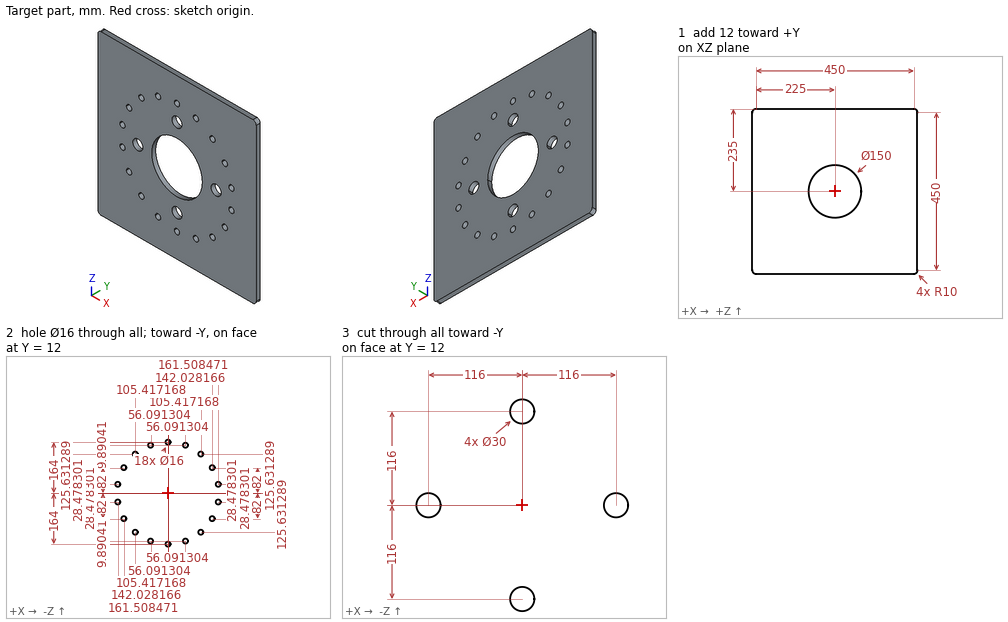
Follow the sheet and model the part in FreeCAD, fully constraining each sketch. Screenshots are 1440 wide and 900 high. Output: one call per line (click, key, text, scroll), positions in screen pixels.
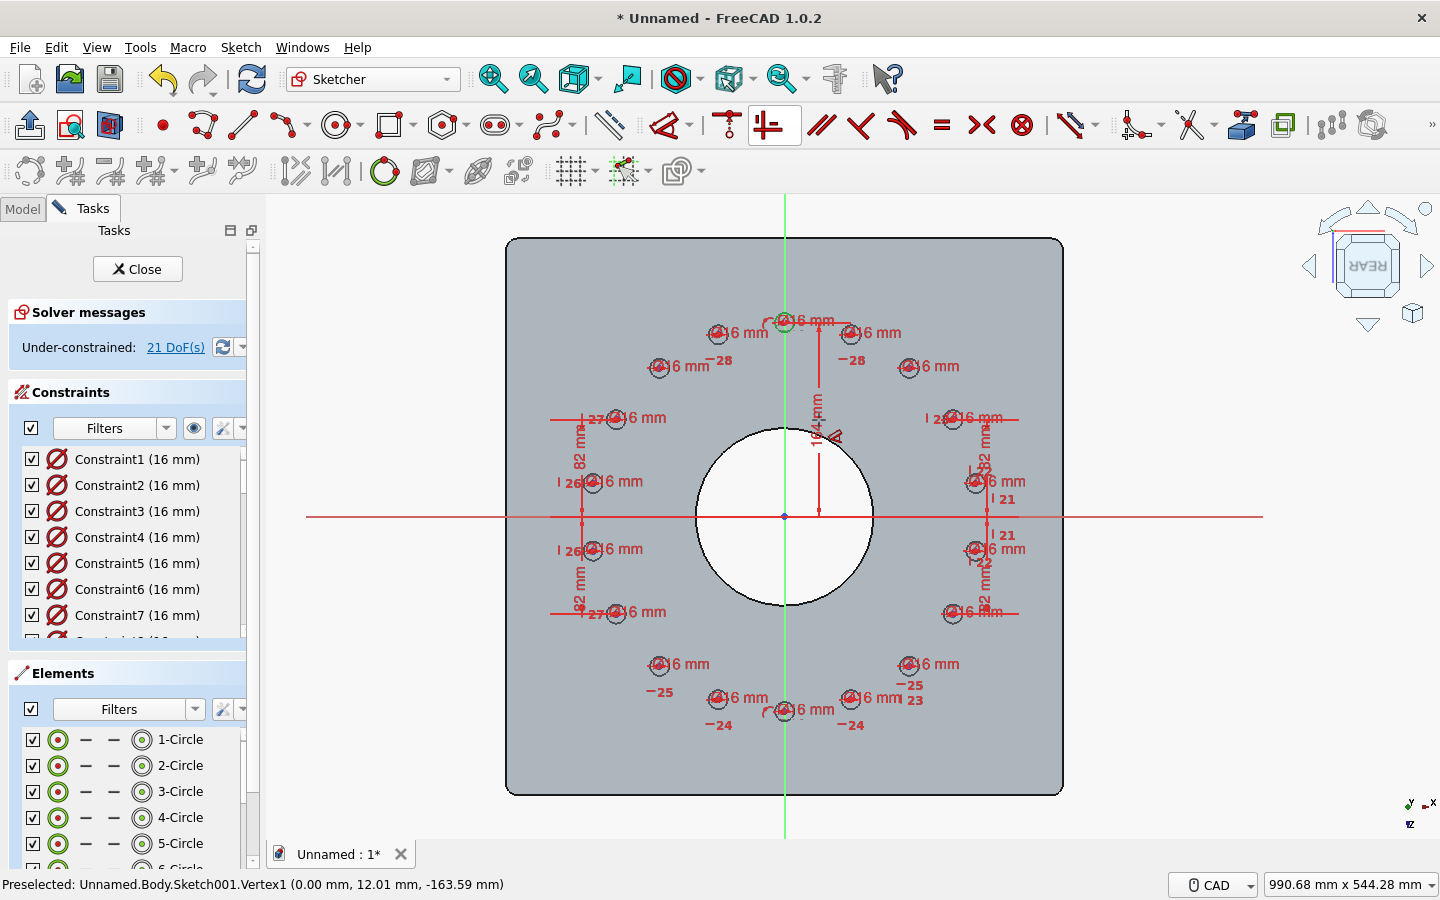
click(785, 712)
click(819, 614)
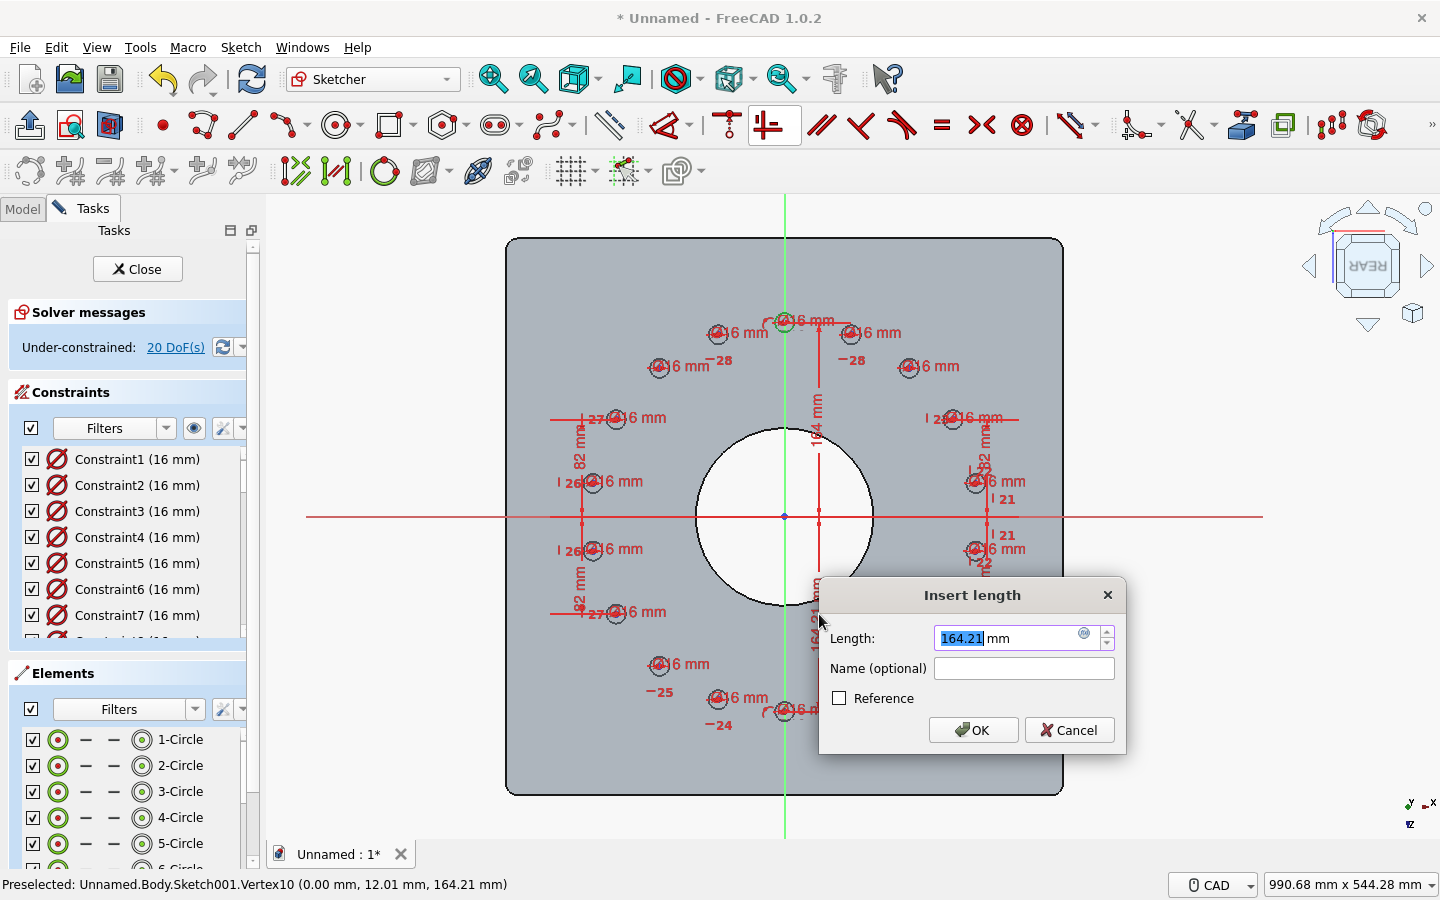
text(164)
key(Return)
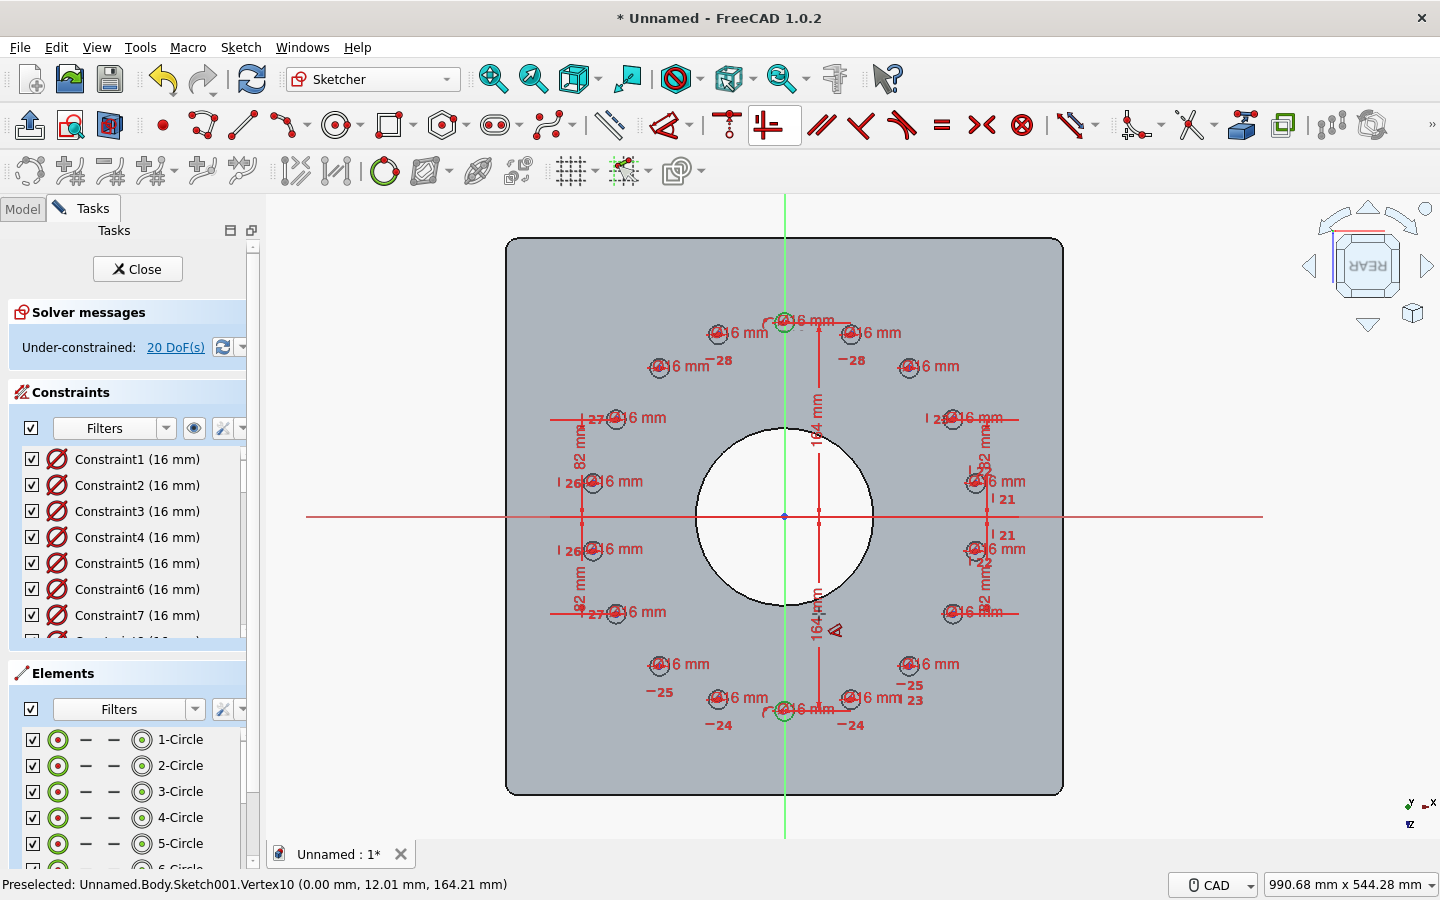
scroll(785, 323, up, 7)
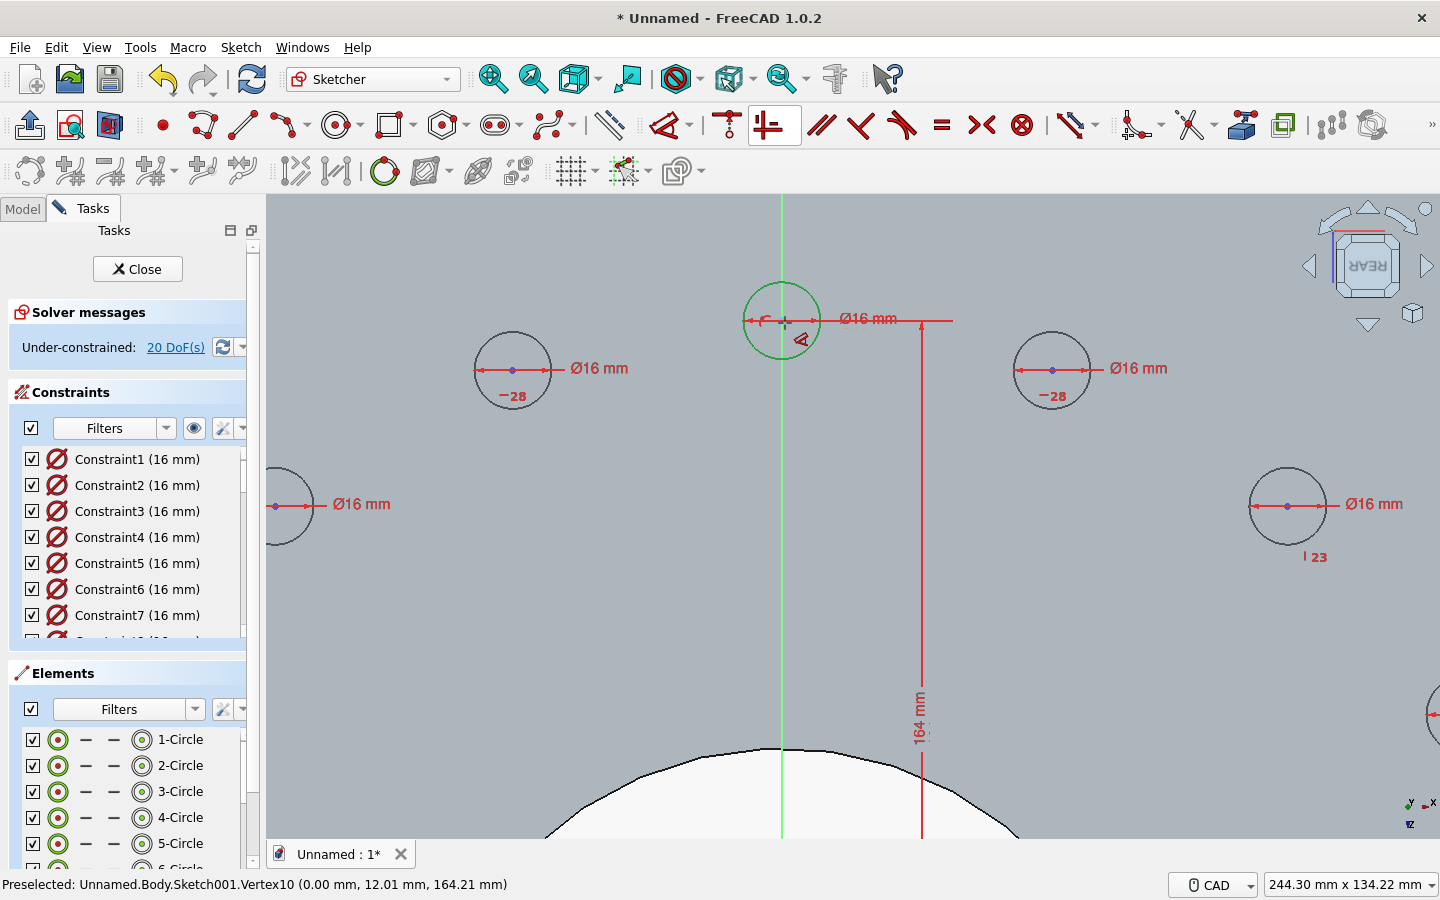
click(782, 321)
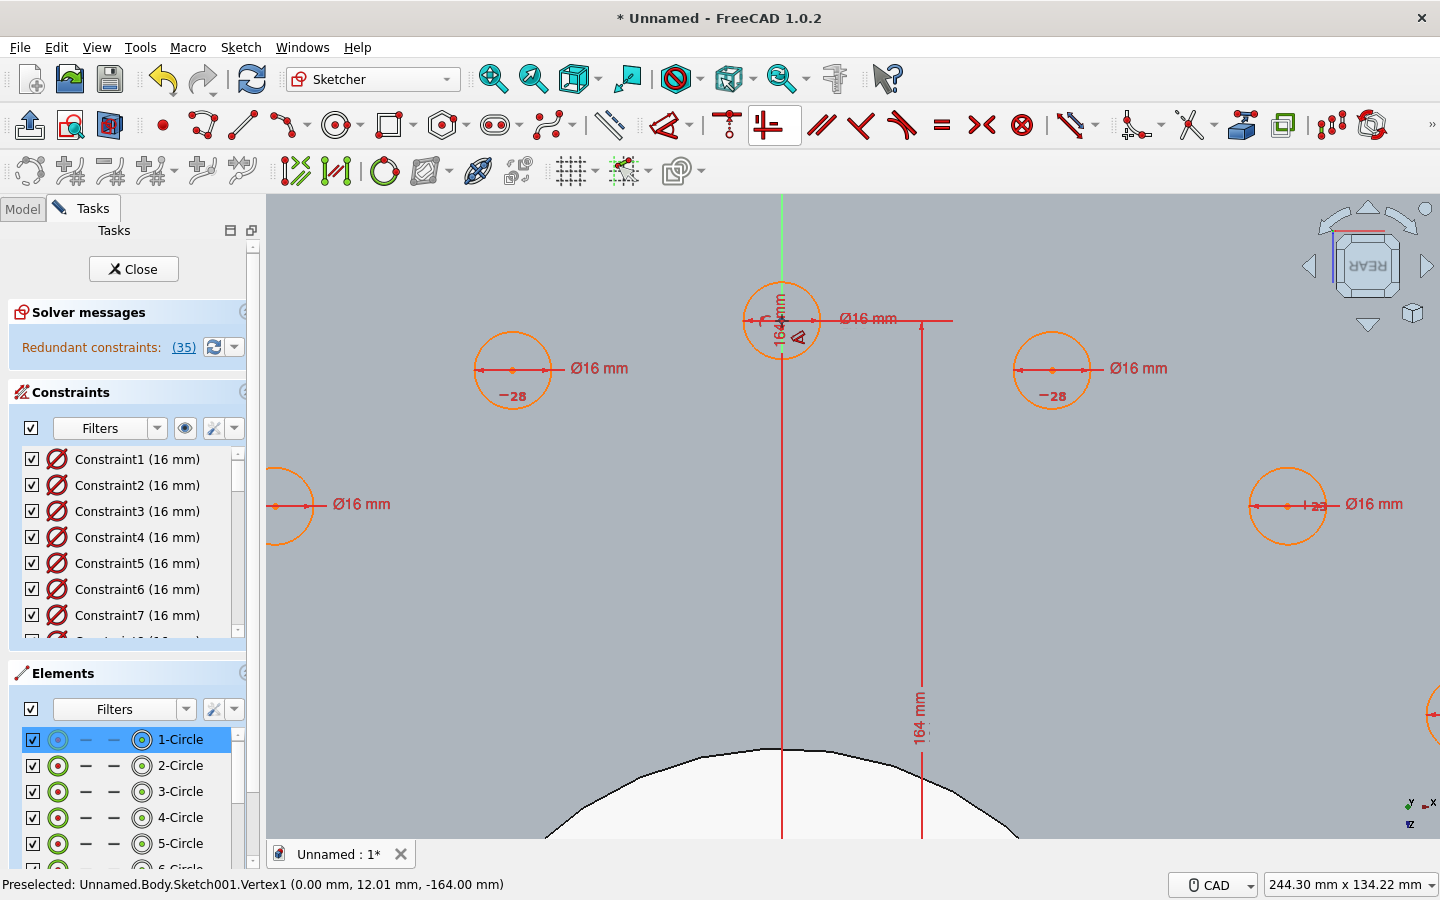
click(1052, 370)
click(1086, 328)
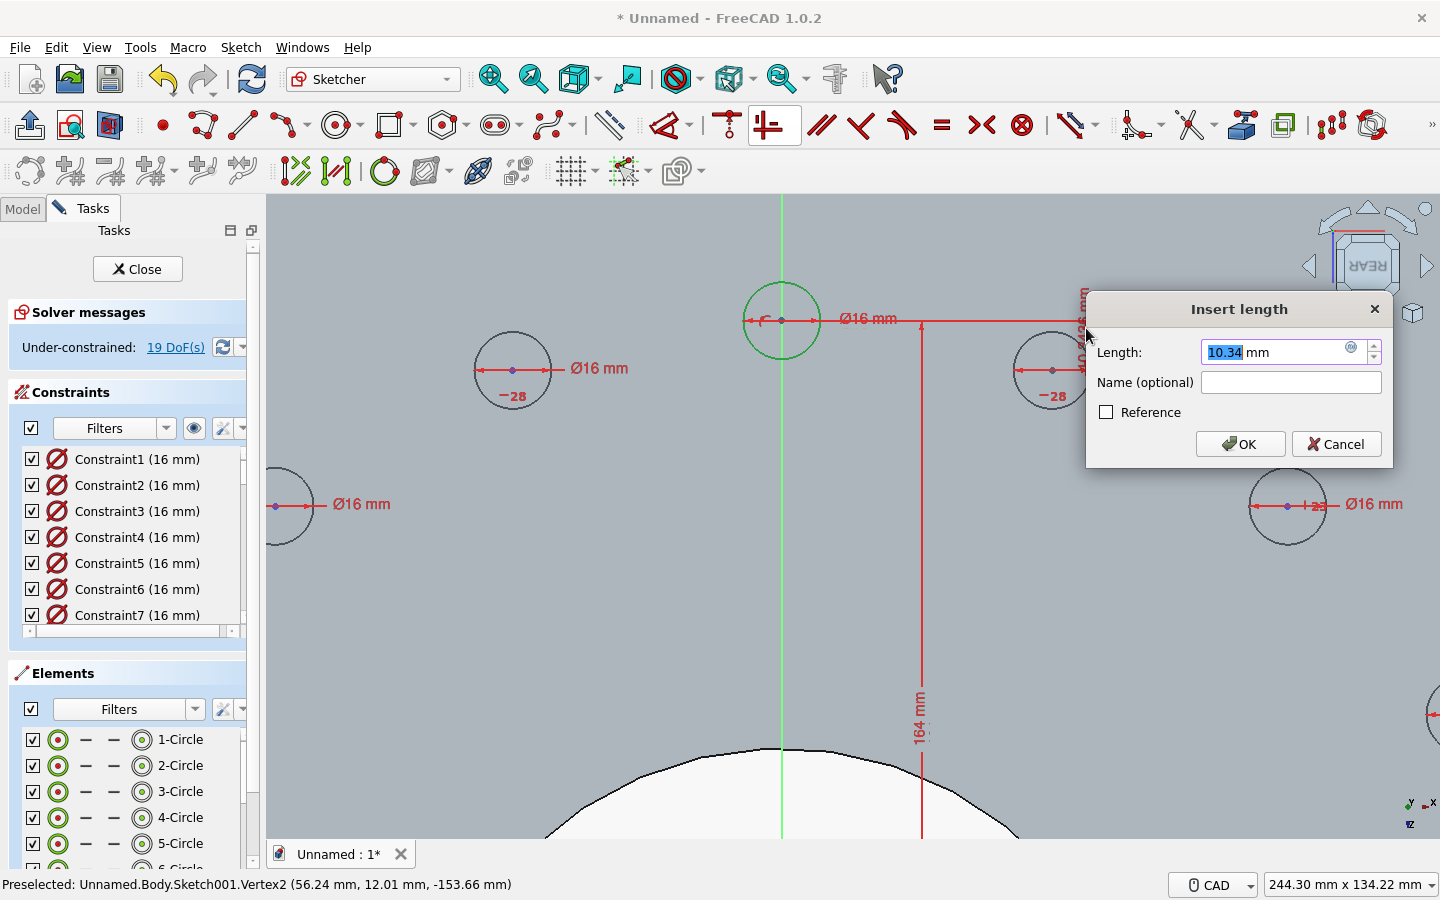
text(9.89041)
key(Return)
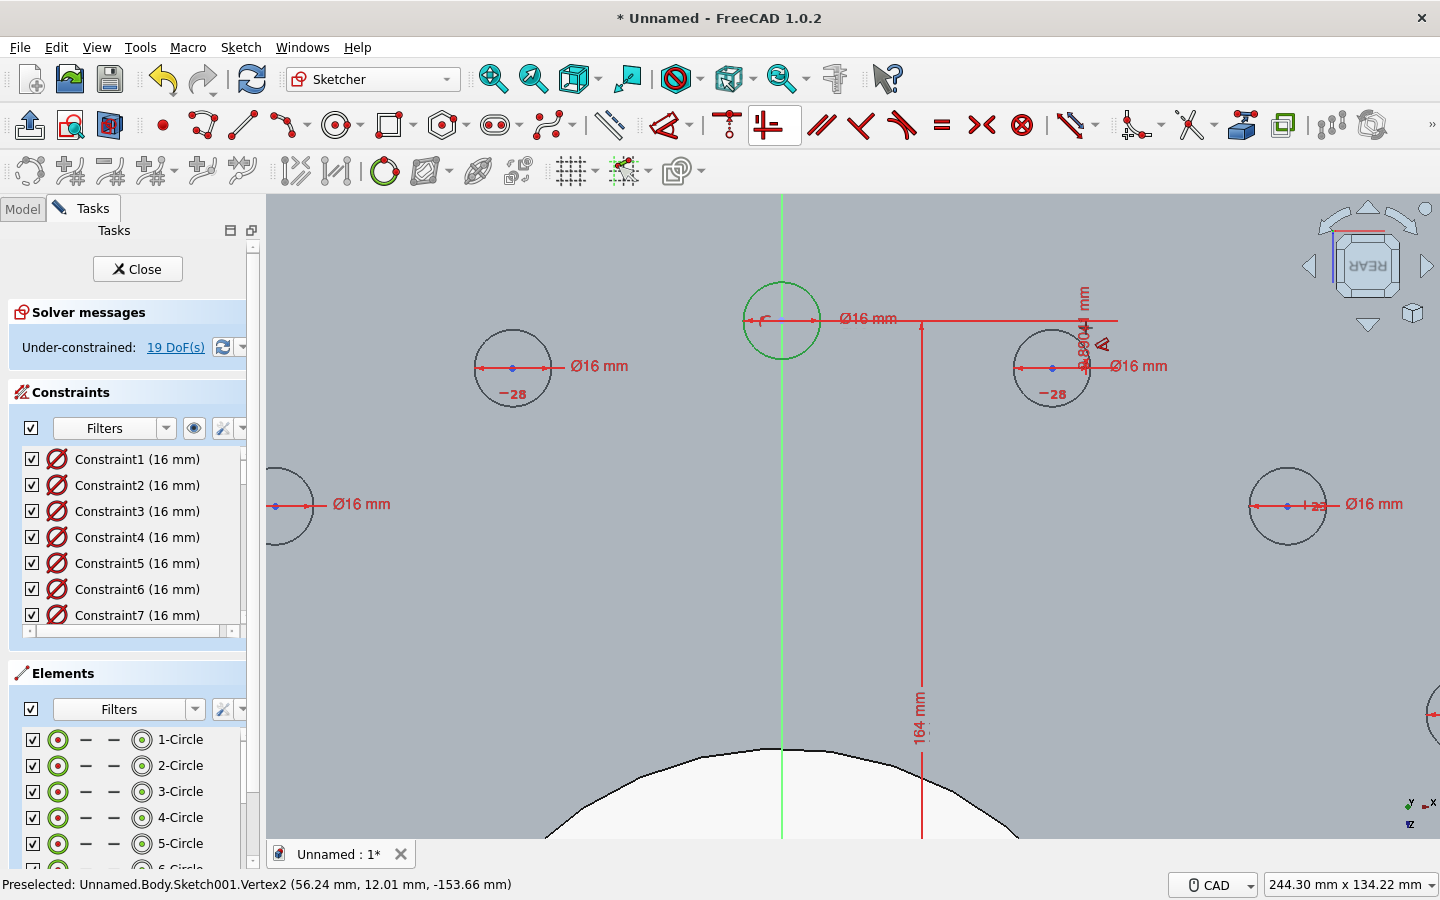
scroll(785, 323, down, 7)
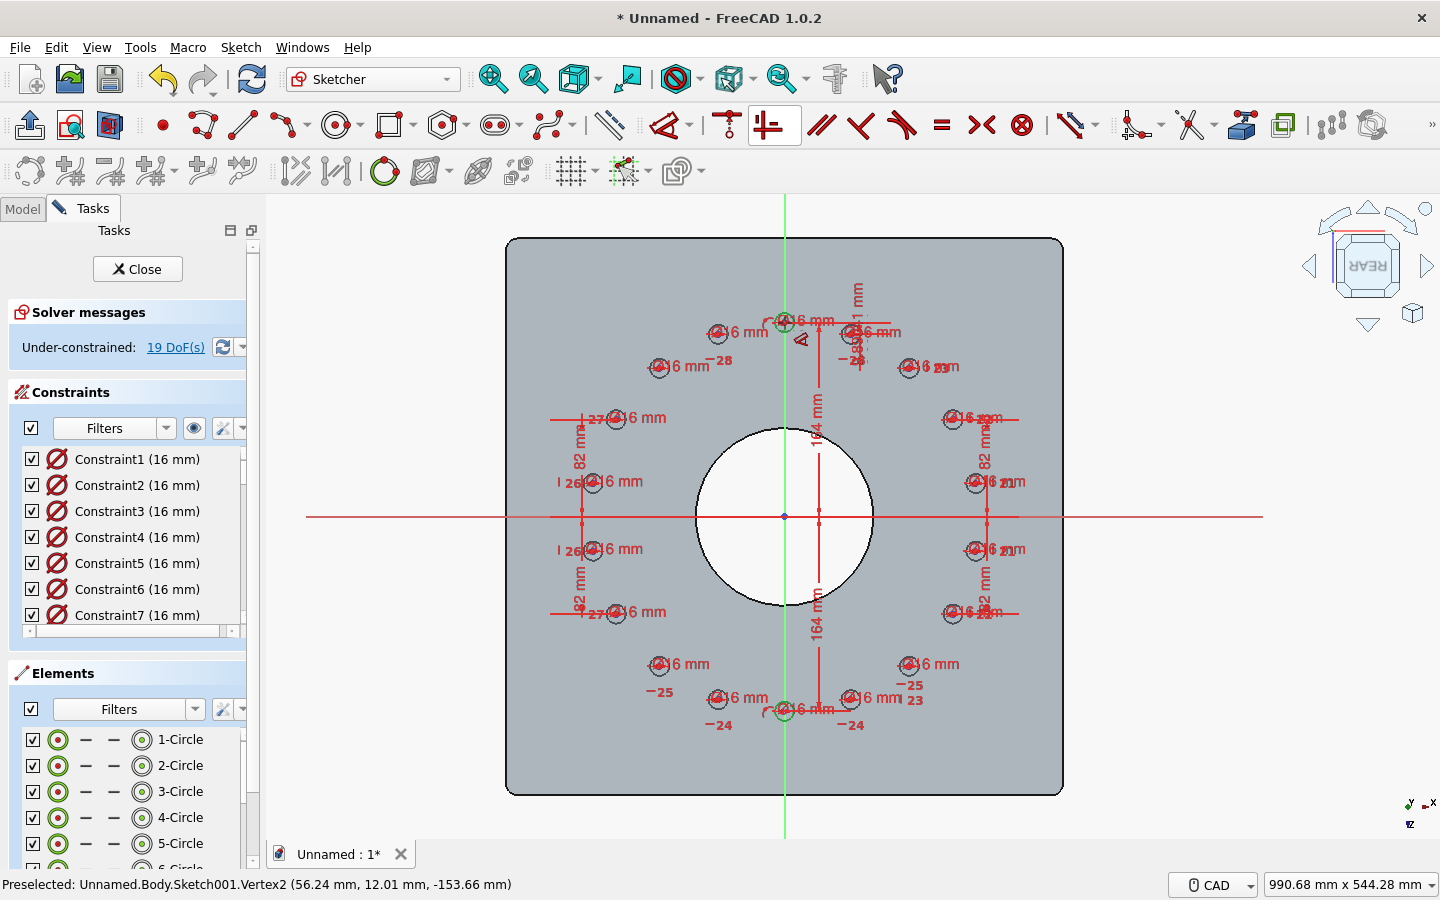
scroll(851, 700, up, 7)